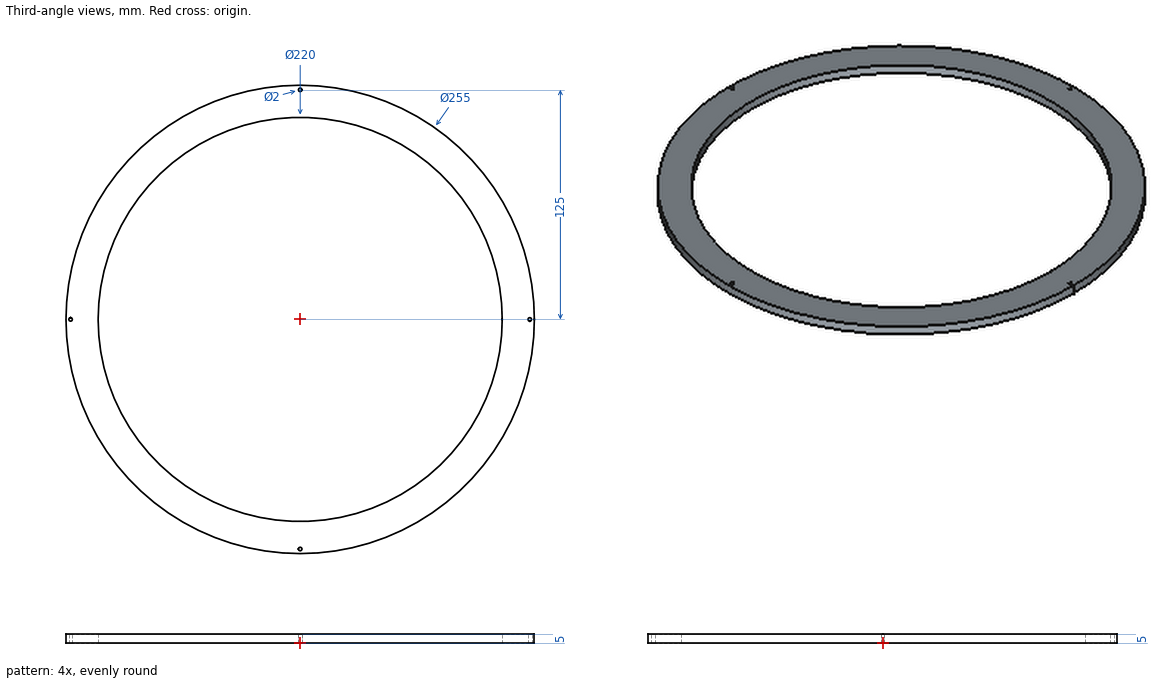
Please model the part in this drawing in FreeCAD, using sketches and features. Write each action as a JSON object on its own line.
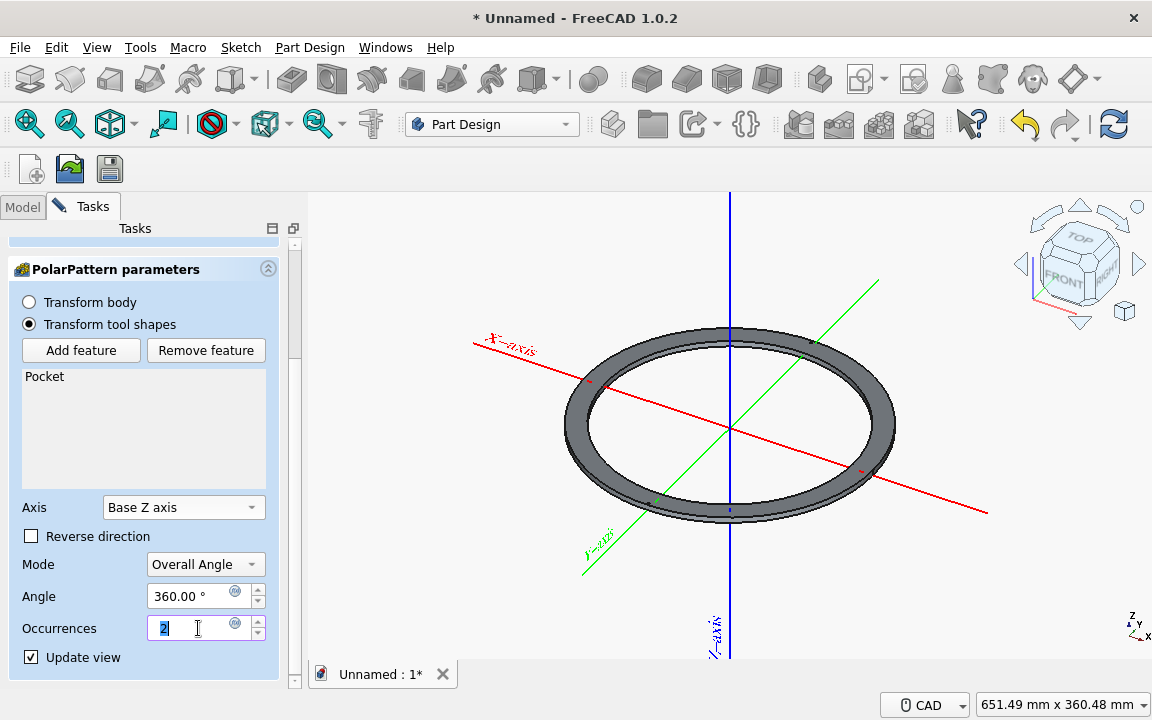
{"action": "type", "text": "4"}
{"action": "key", "text": "Tab"}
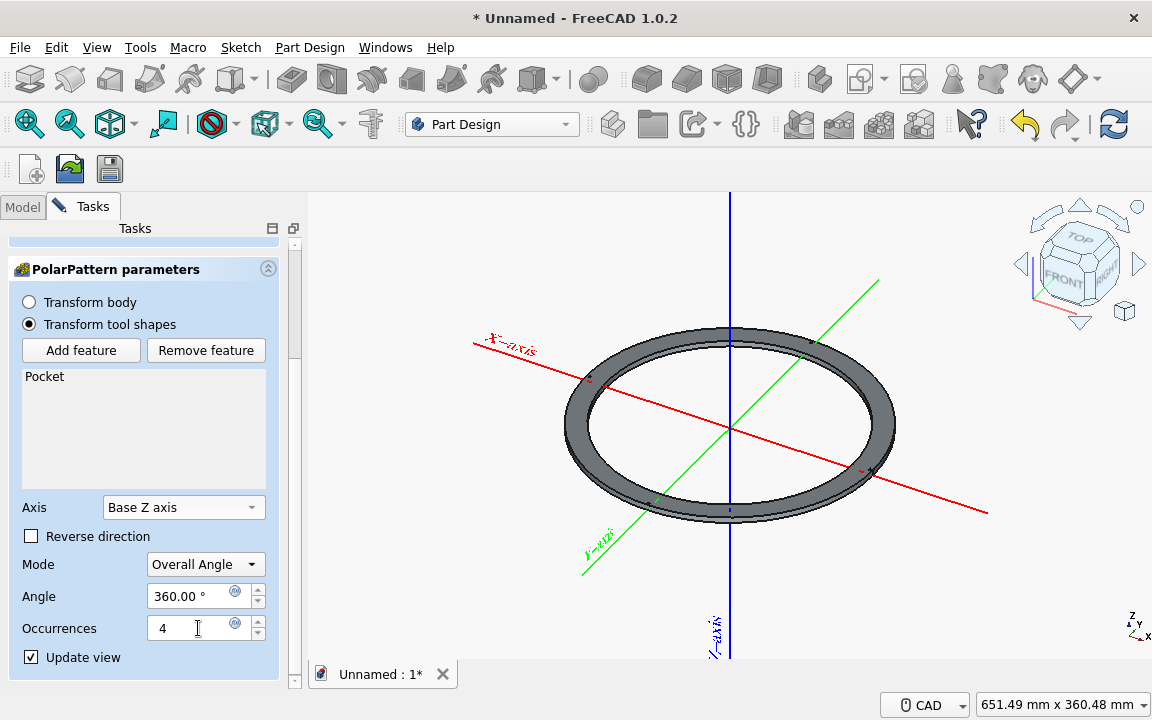
{"action": "scroll", "coordinate": [295, 463], "scroll_direction": "up", "scroll_amount": 4}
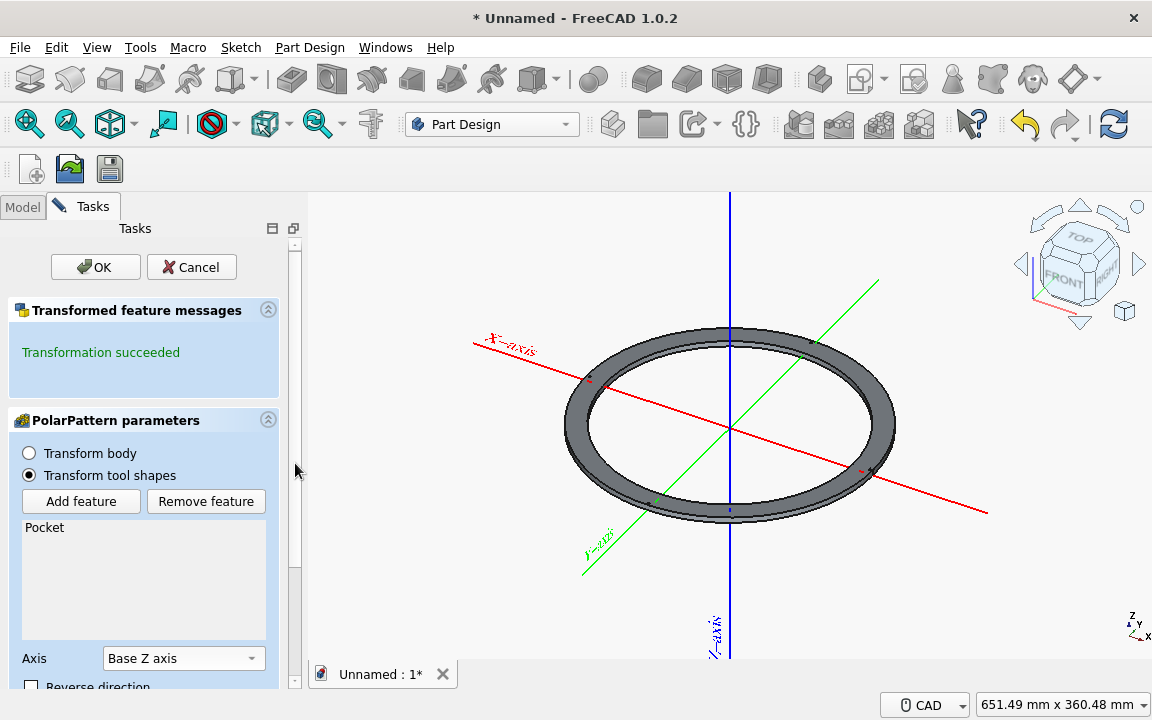
{"action": "left_click", "coordinate": [96, 267]}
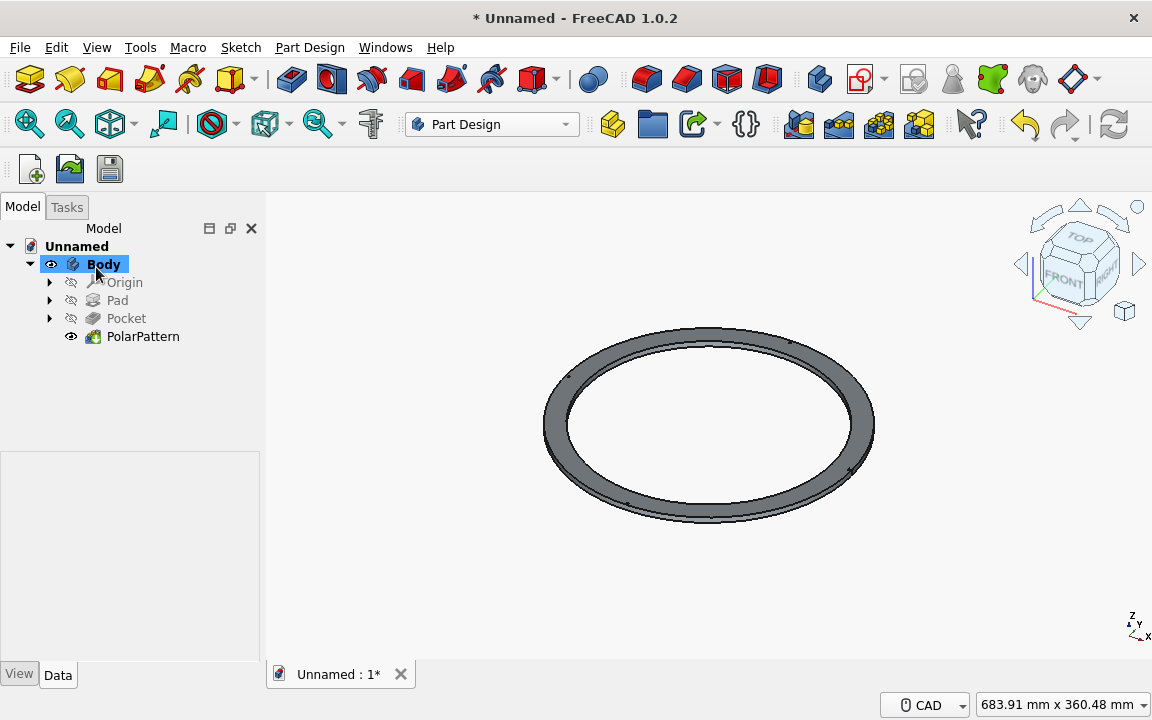
{"action": "key", "text": "0"}